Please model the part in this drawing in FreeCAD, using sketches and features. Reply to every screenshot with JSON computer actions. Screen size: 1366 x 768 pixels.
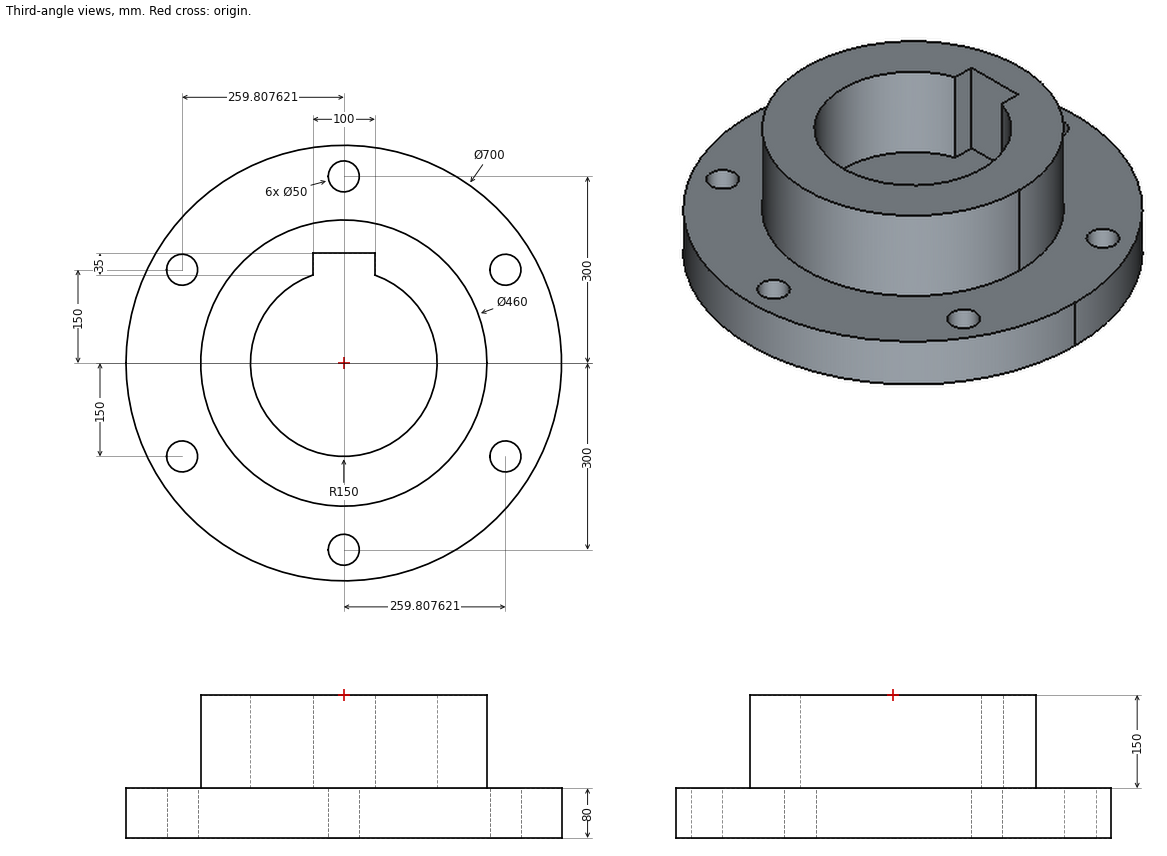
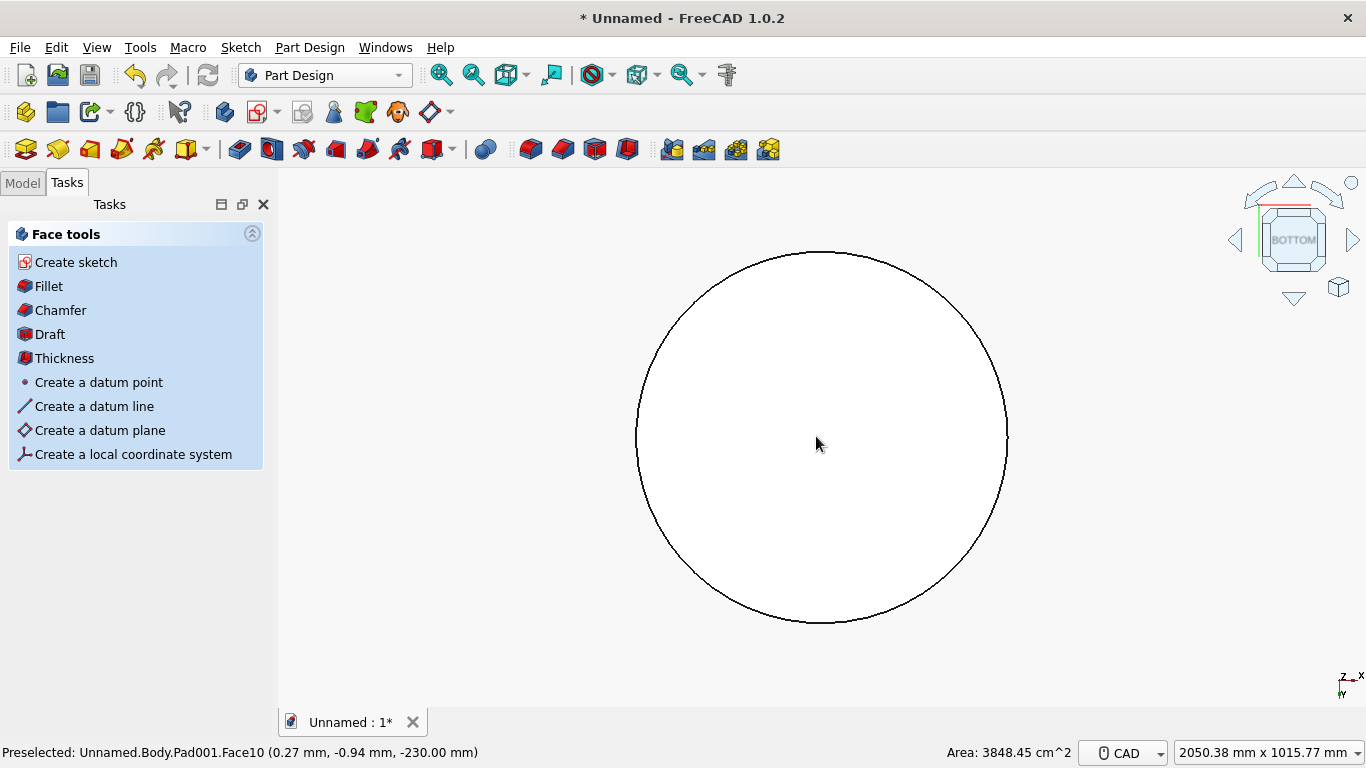
{"action": "left_click", "coordinate": [258, 112]}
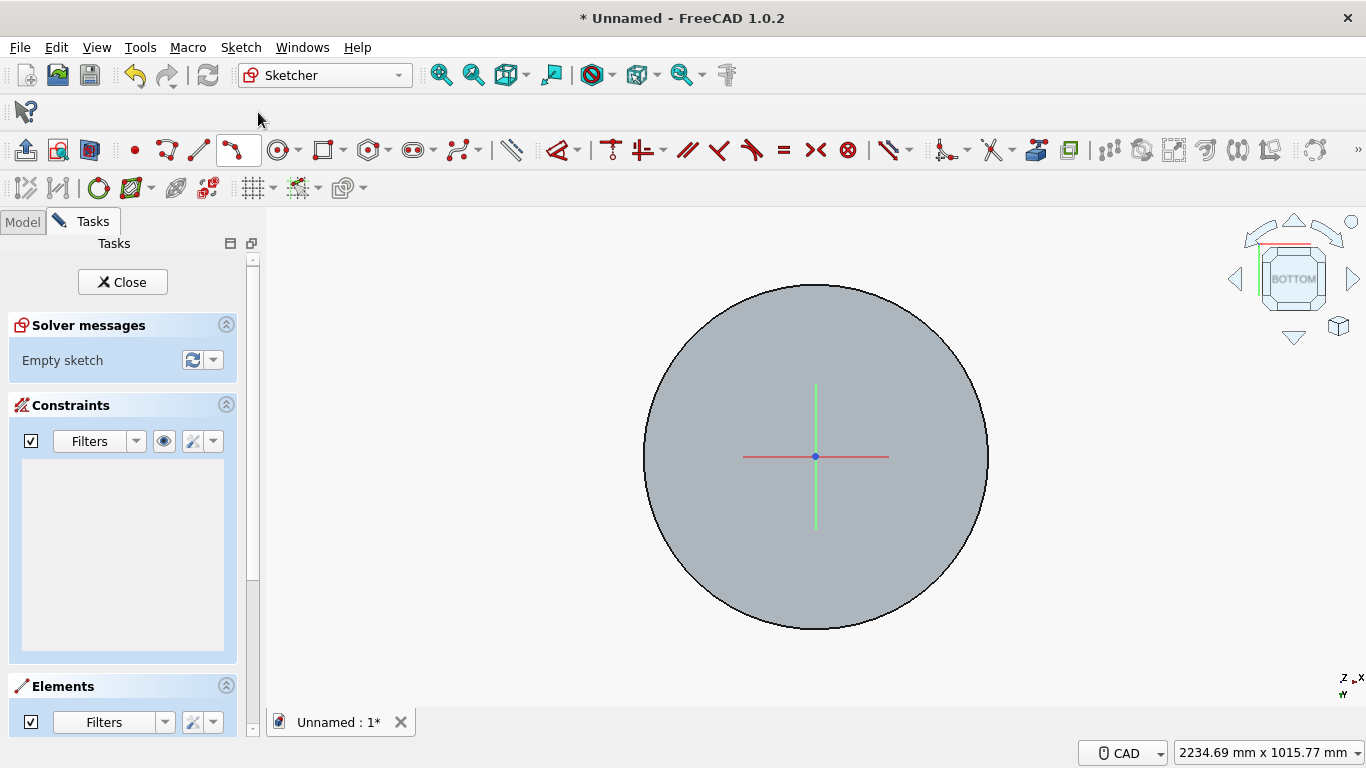
{"action": "left_click", "coordinate": [278, 150]}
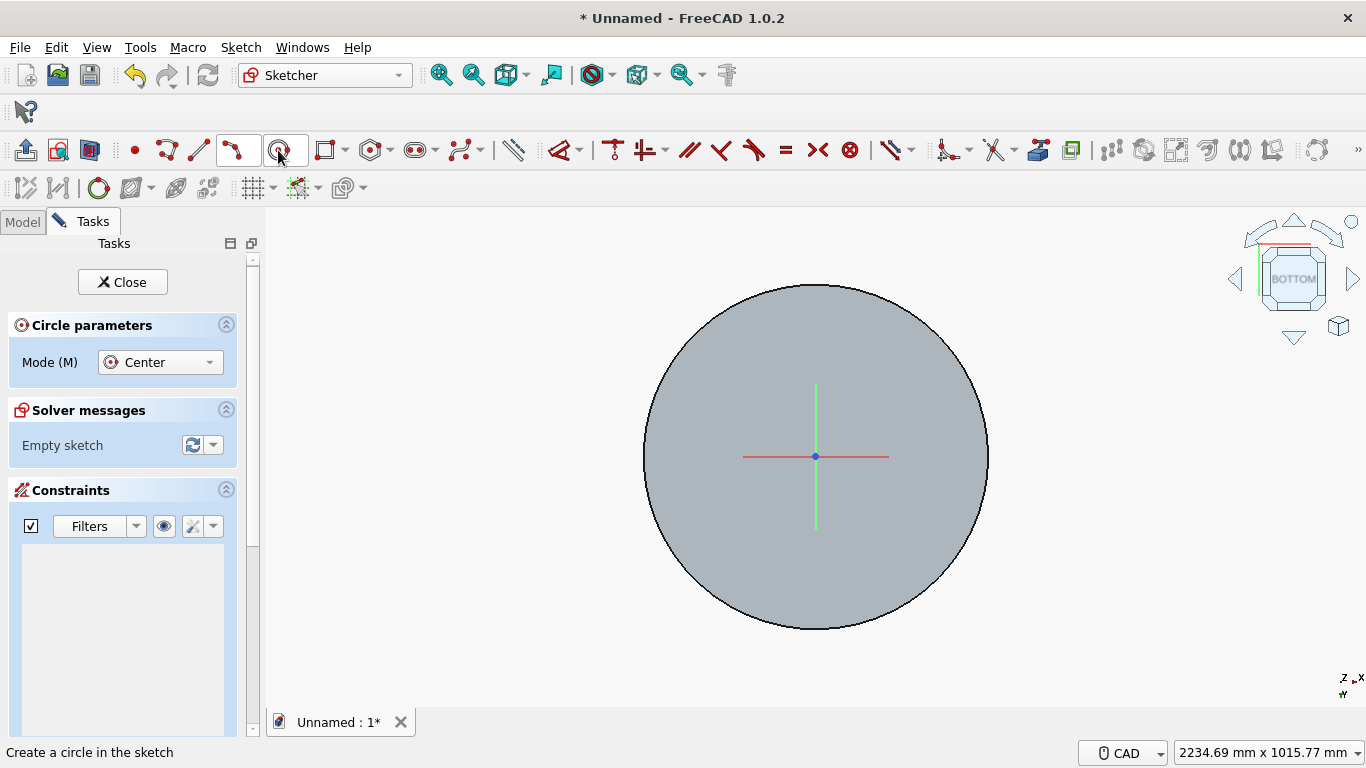
{"action": "scroll", "coordinate": [816, 605], "scroll_direction": "up", "scroll_amount": 4}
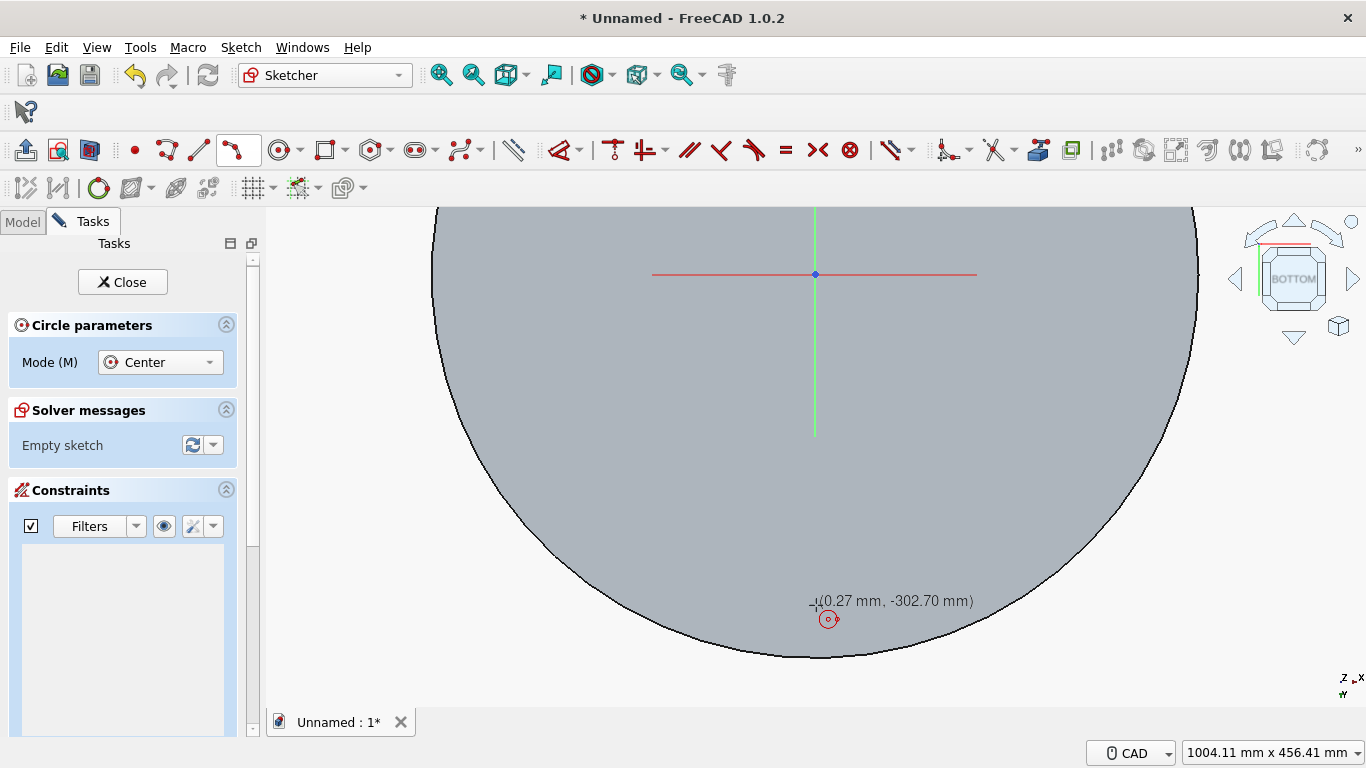
{"action": "left_click", "coordinate": [815, 603]}
{"action": "mouse_move", "coordinate": [834, 584]}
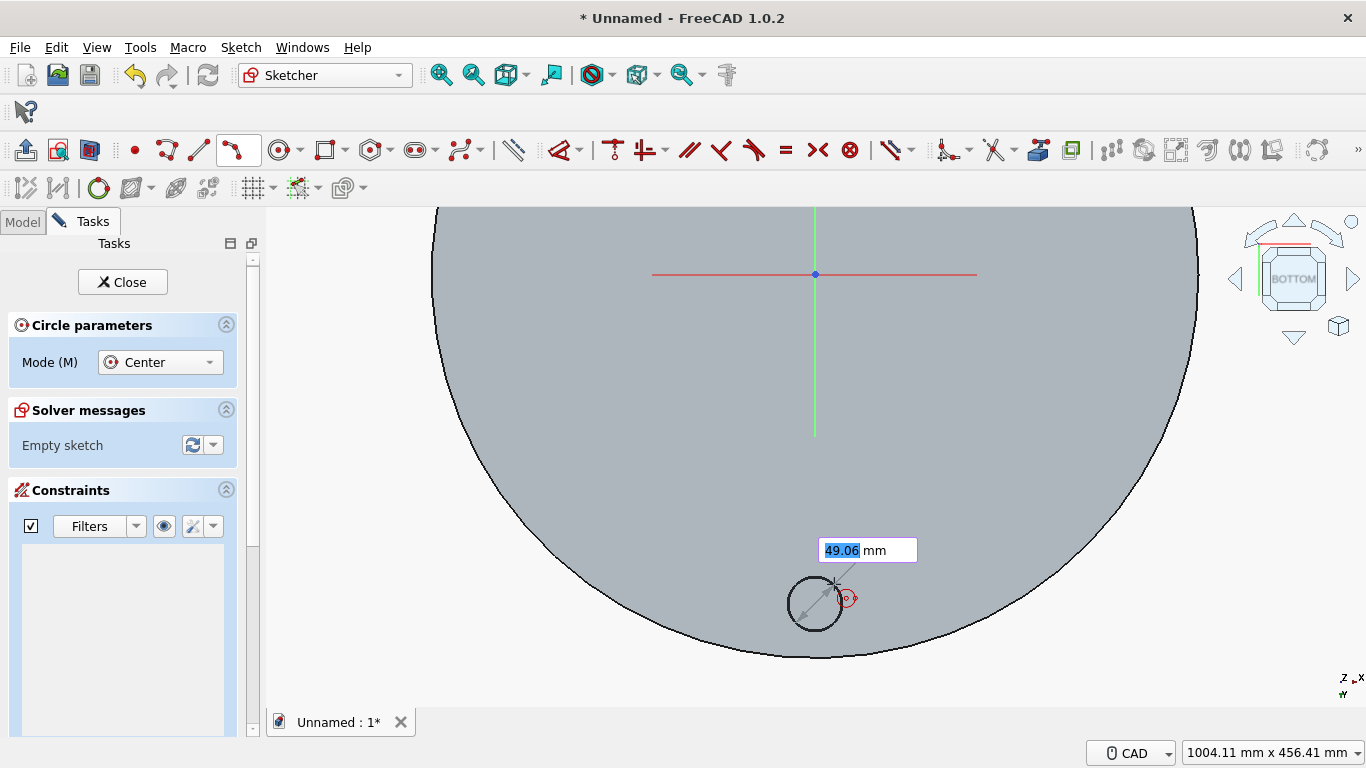
{"action": "type", "text": "50"}
{"action": "key", "text": "Return"}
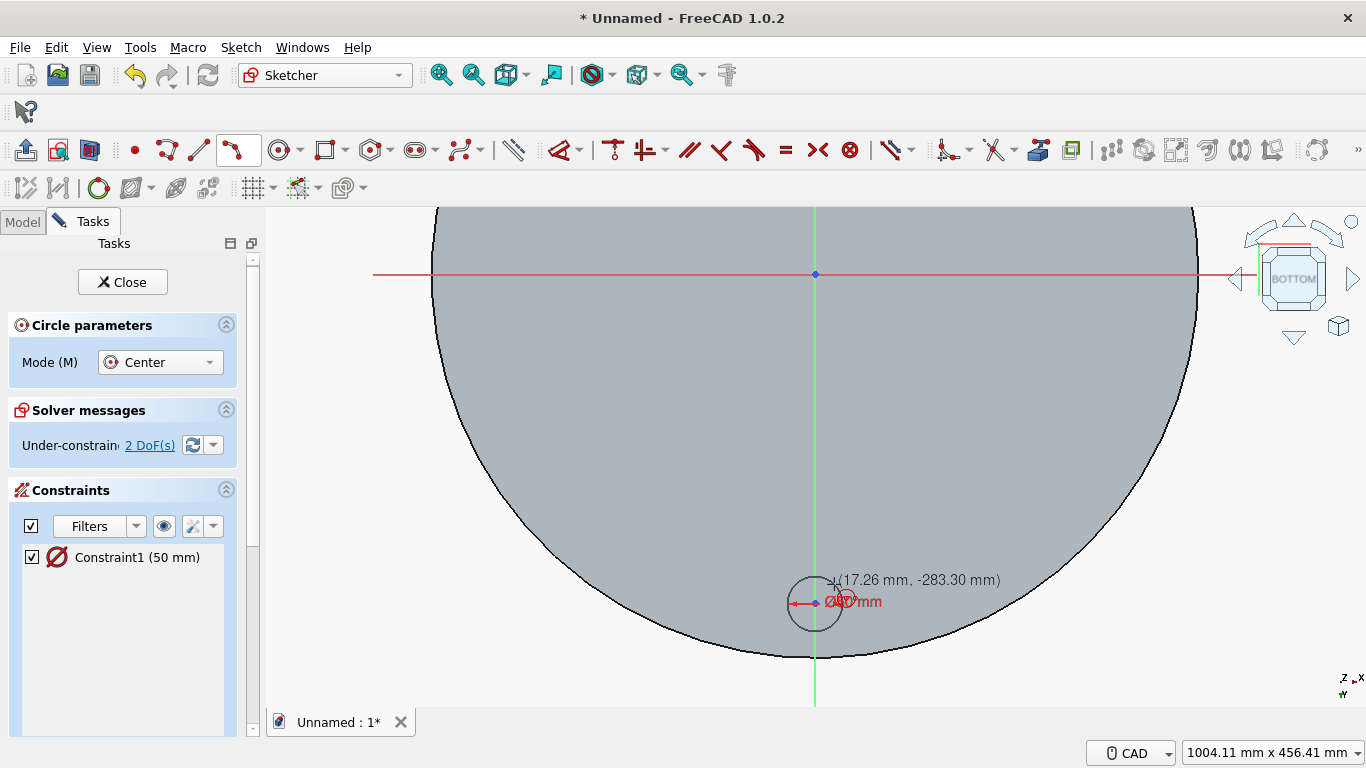
{"action": "left_click", "coordinate": [530, 439]}
{"action": "mouse_move", "coordinate": [550, 420]}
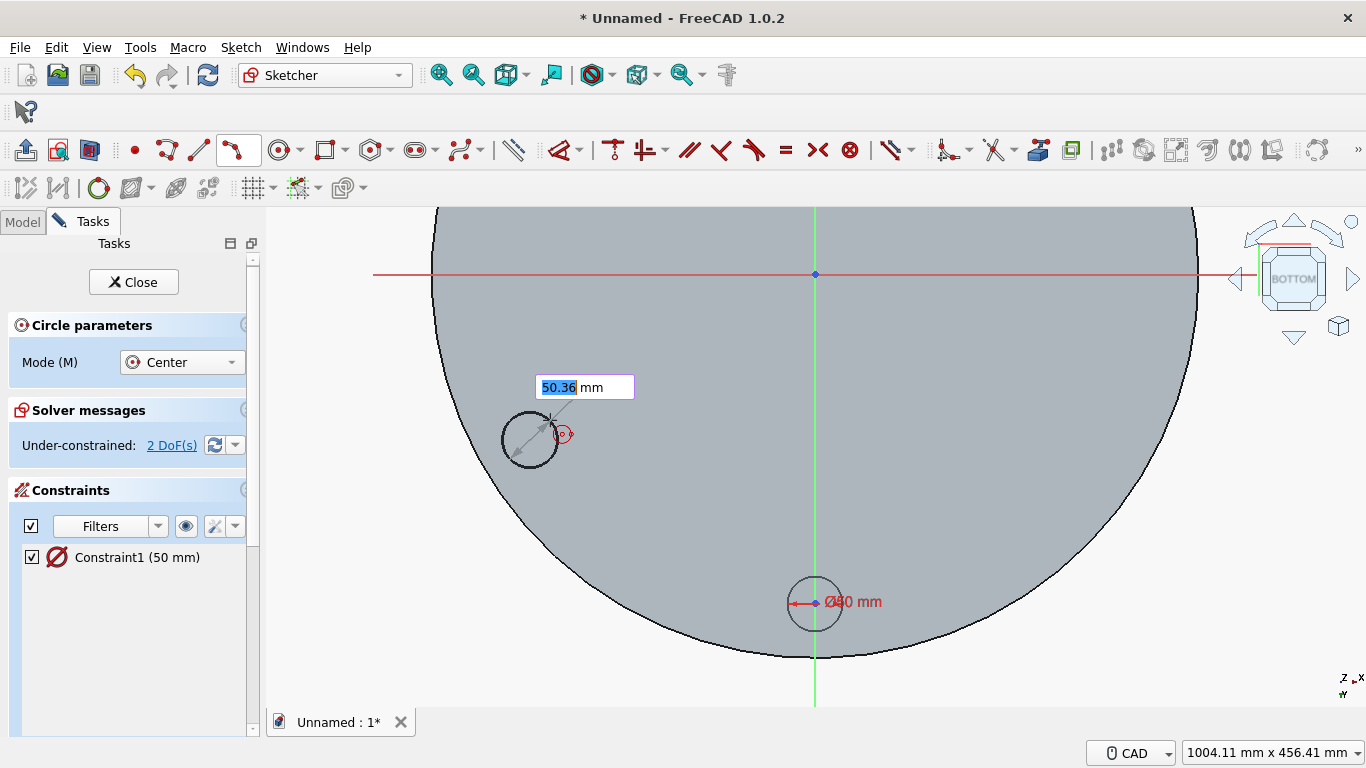
{"action": "type", "text": "50"}
{"action": "key", "text": "Return"}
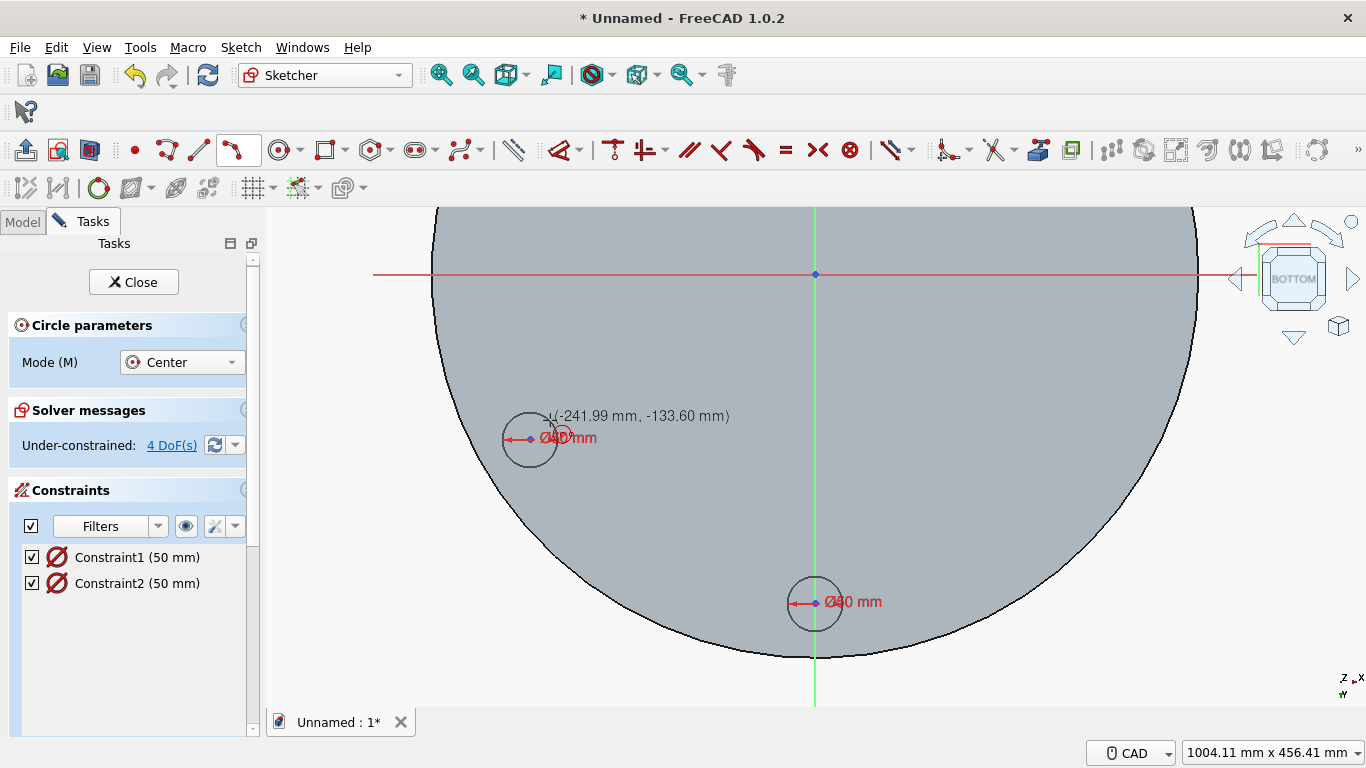
{"action": "scroll", "coordinate": [692, 606], "scroll_direction": "down", "scroll_amount": 4}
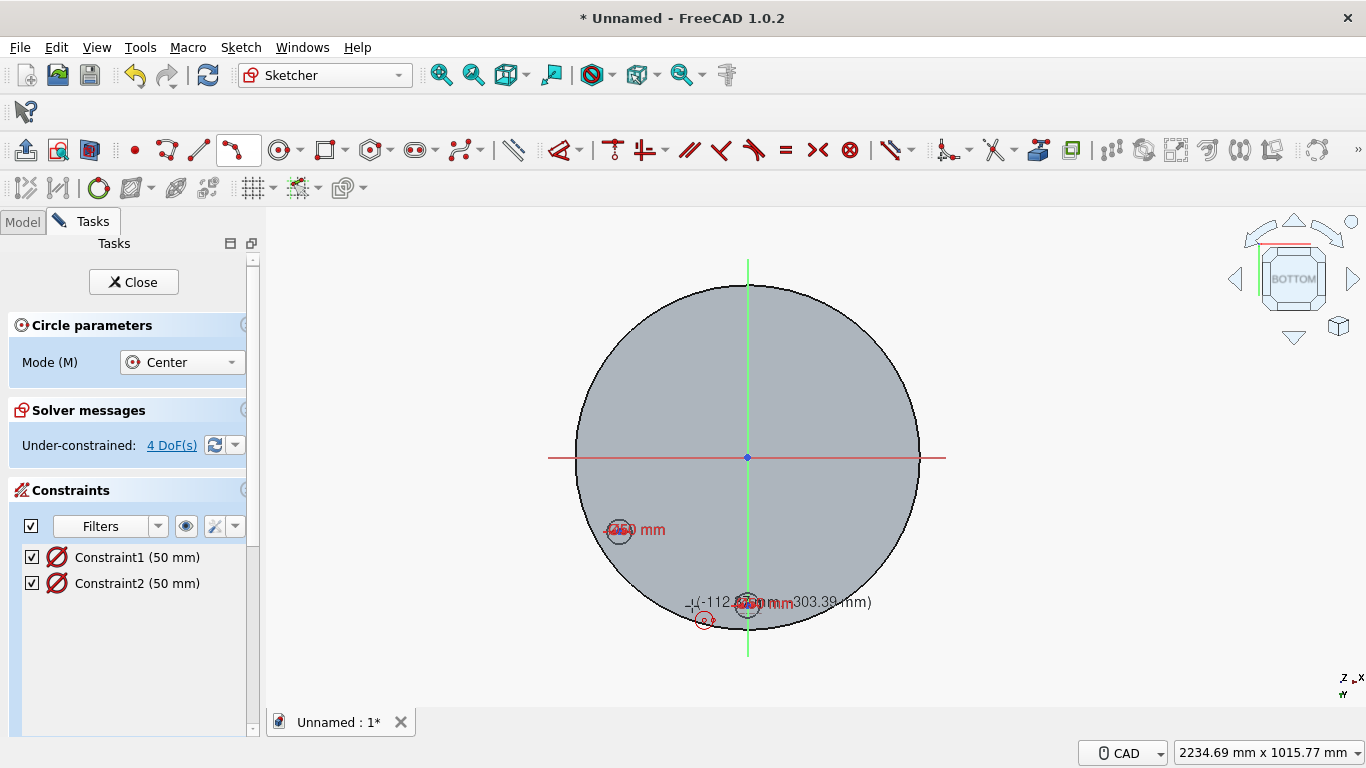
{"action": "scroll", "coordinate": [620, 384], "scroll_direction": "up", "scroll_amount": 4}